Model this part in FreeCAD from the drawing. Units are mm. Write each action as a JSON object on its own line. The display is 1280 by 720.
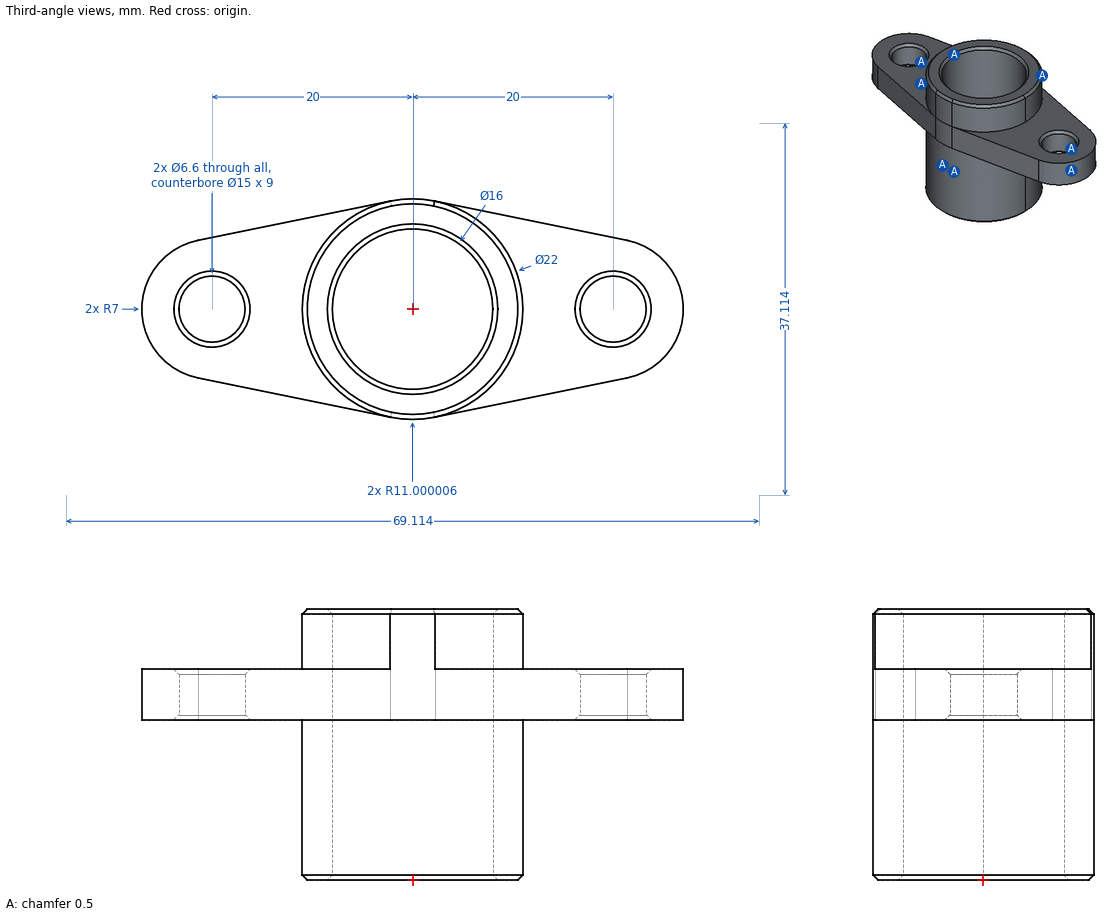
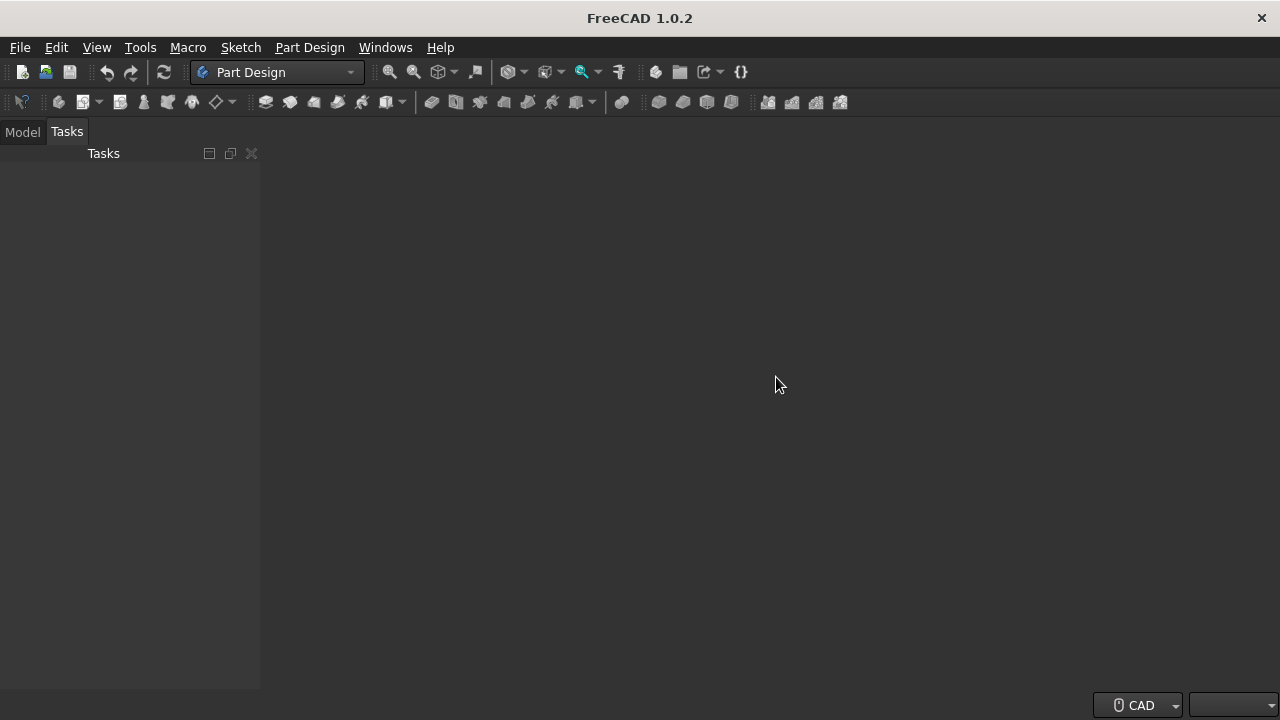
{"action": "left_click", "coordinate": [22, 72]}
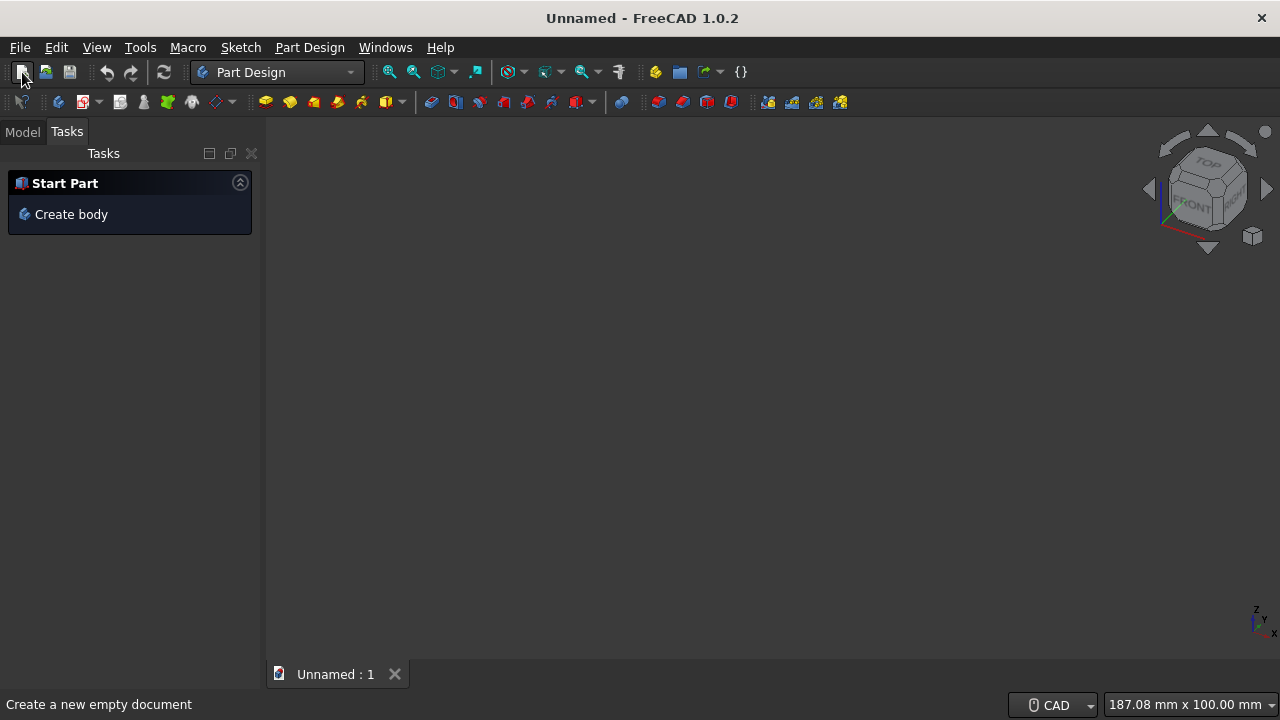
{"action": "left_click", "coordinate": [84, 102]}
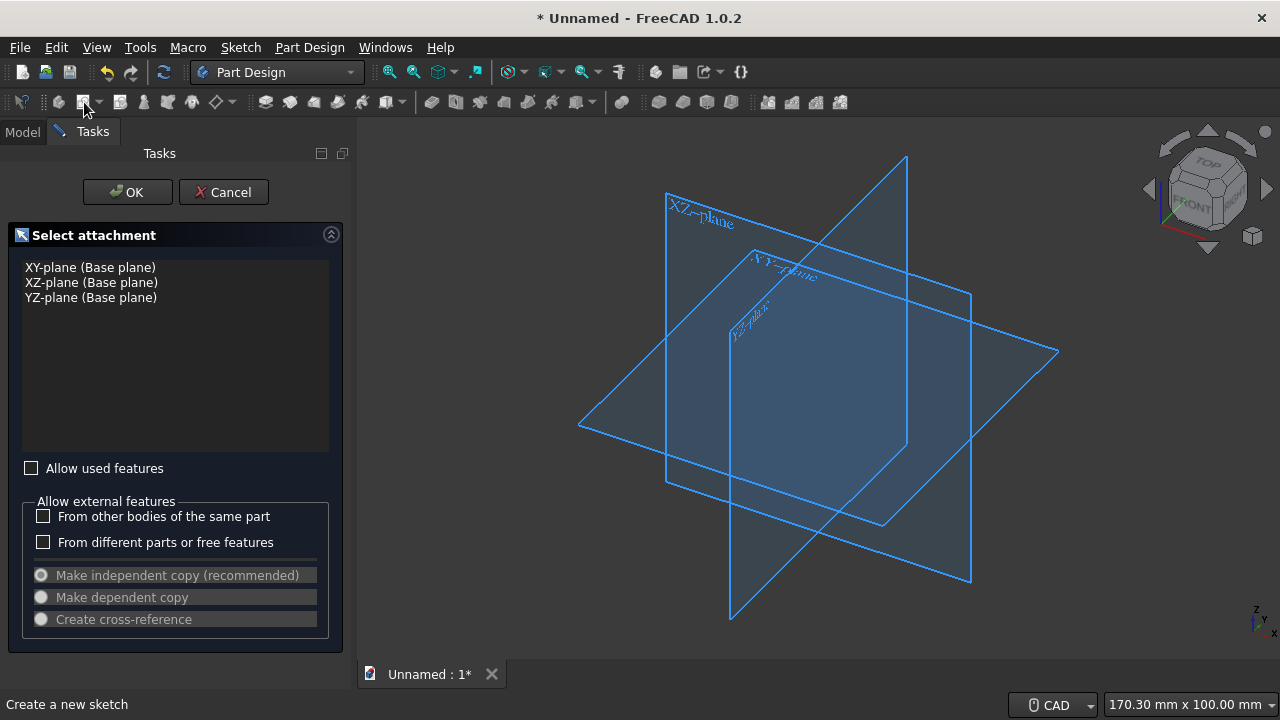
{"action": "left_click", "coordinate": [82, 268]}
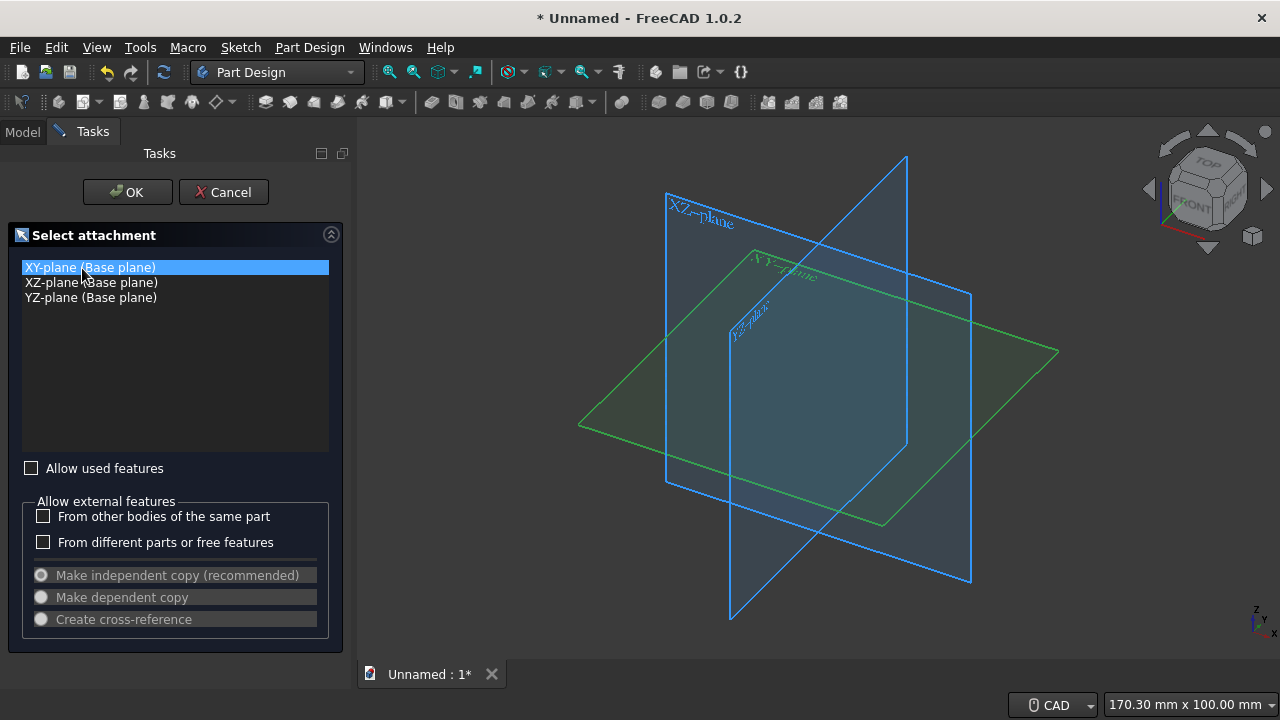
{"action": "left_click", "coordinate": [128, 192]}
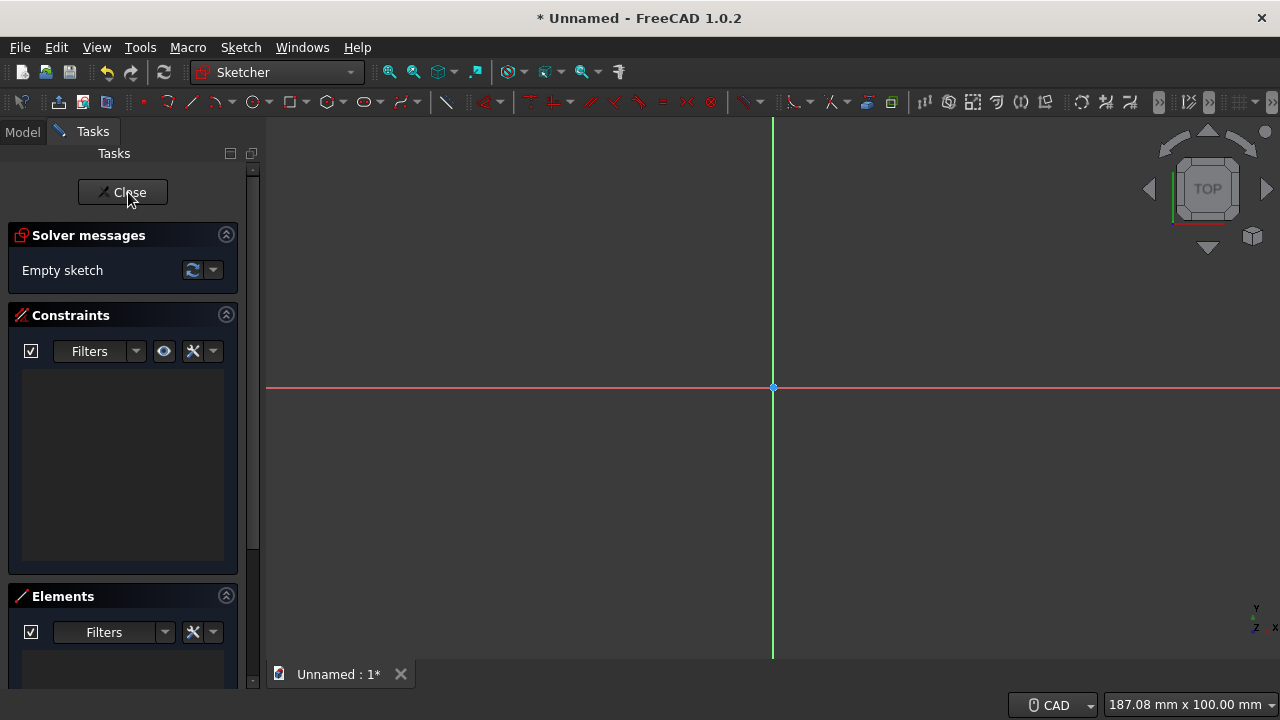
{"action": "scroll", "coordinate": [813, 388], "scroll_direction": "up", "scroll_amount": 5}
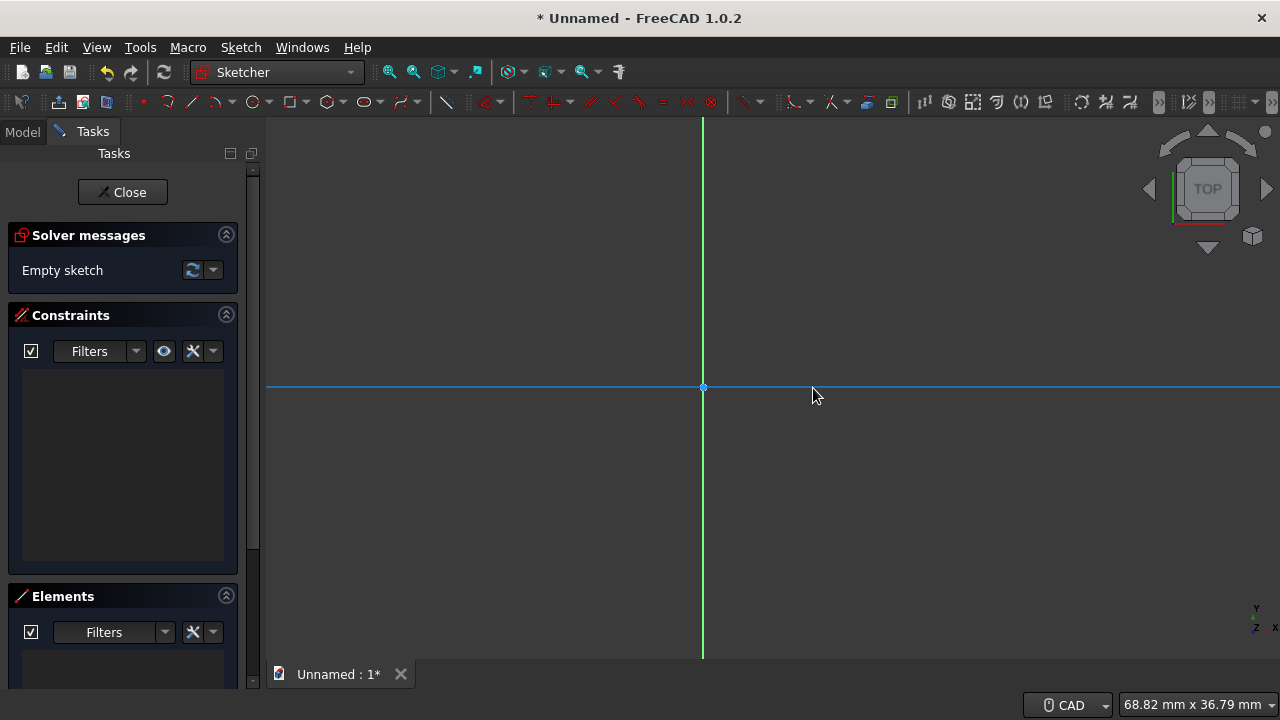
{"action": "left_click", "coordinate": [254, 102]}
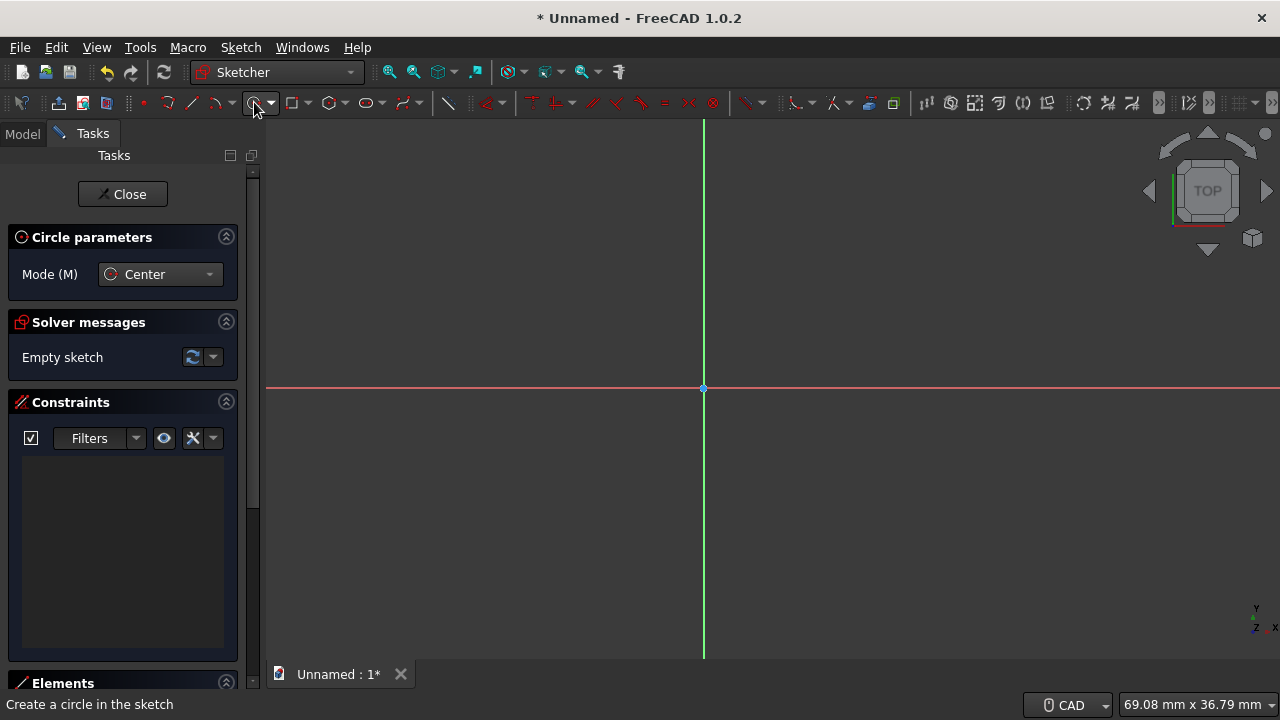
{"action": "left_click", "coordinate": [704, 388]}
{"action": "left_click", "coordinate": [818, 274]}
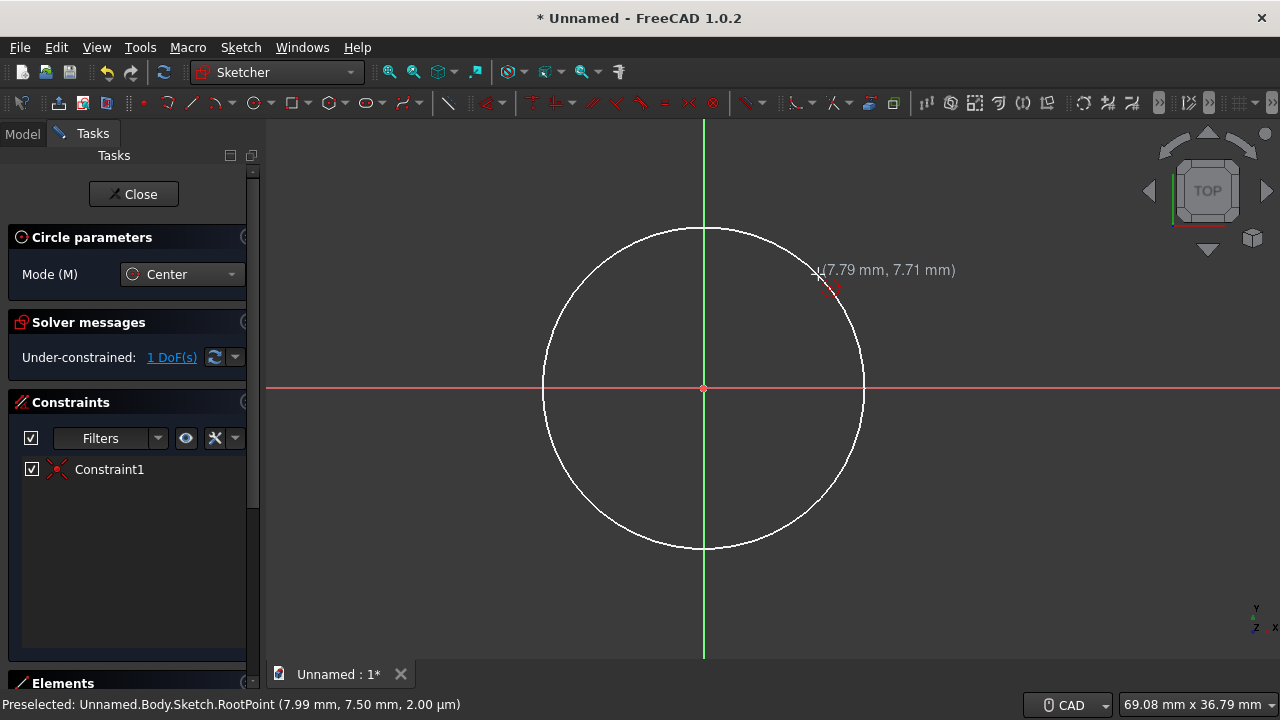
{"action": "left_click", "coordinate": [704, 388]}
{"action": "left_click", "coordinate": [787, 305]}
{"action": "key", "text": "Escape"}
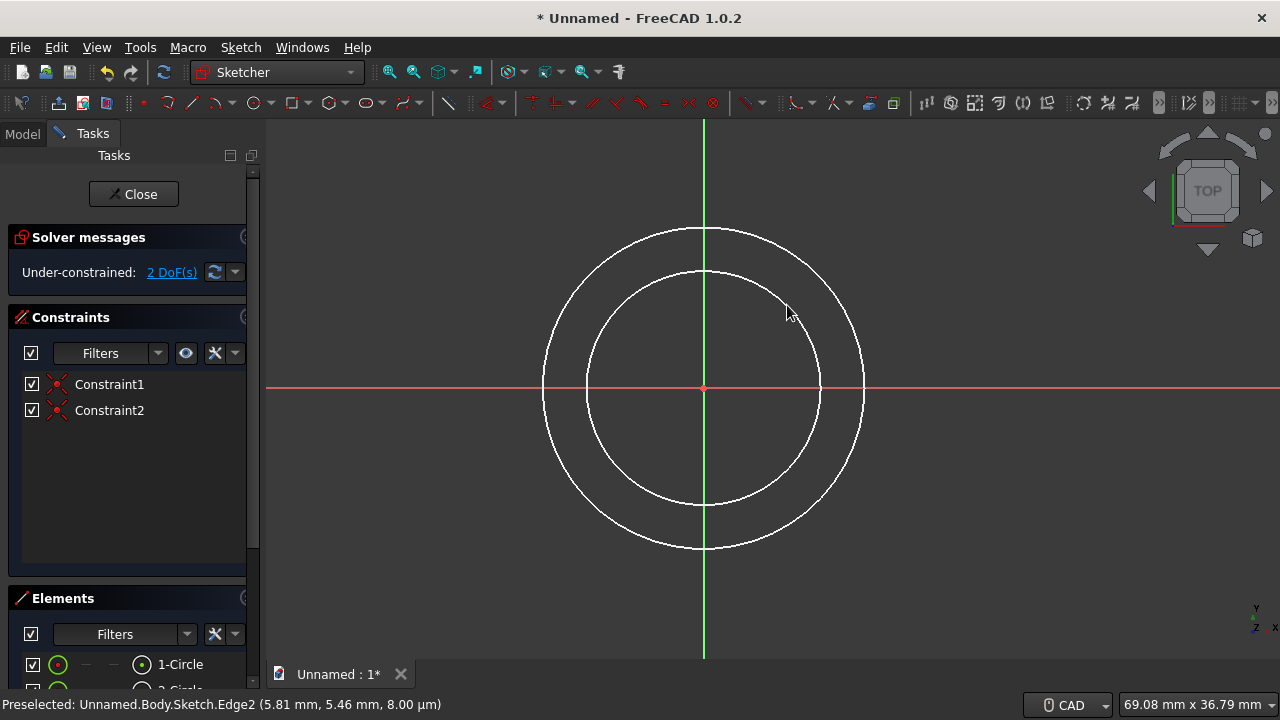
{"action": "left_click", "coordinate": [817, 274]}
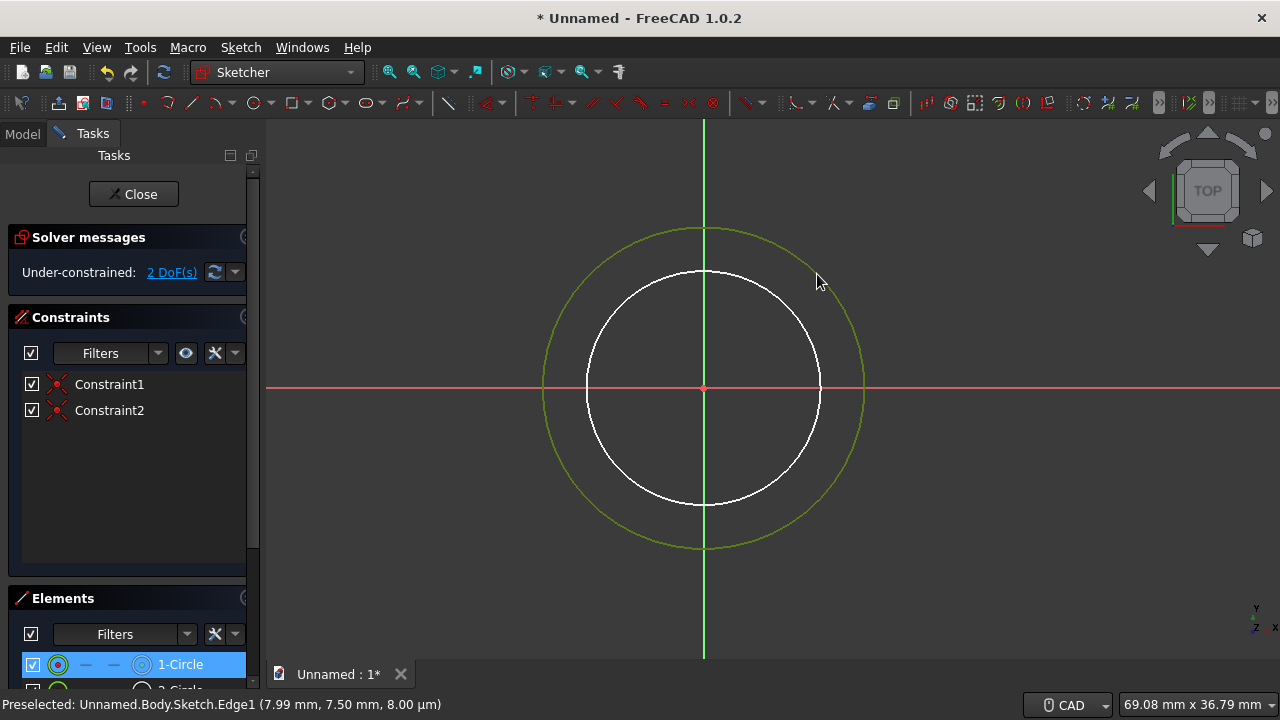
{"action": "left_click", "coordinate": [504, 104]}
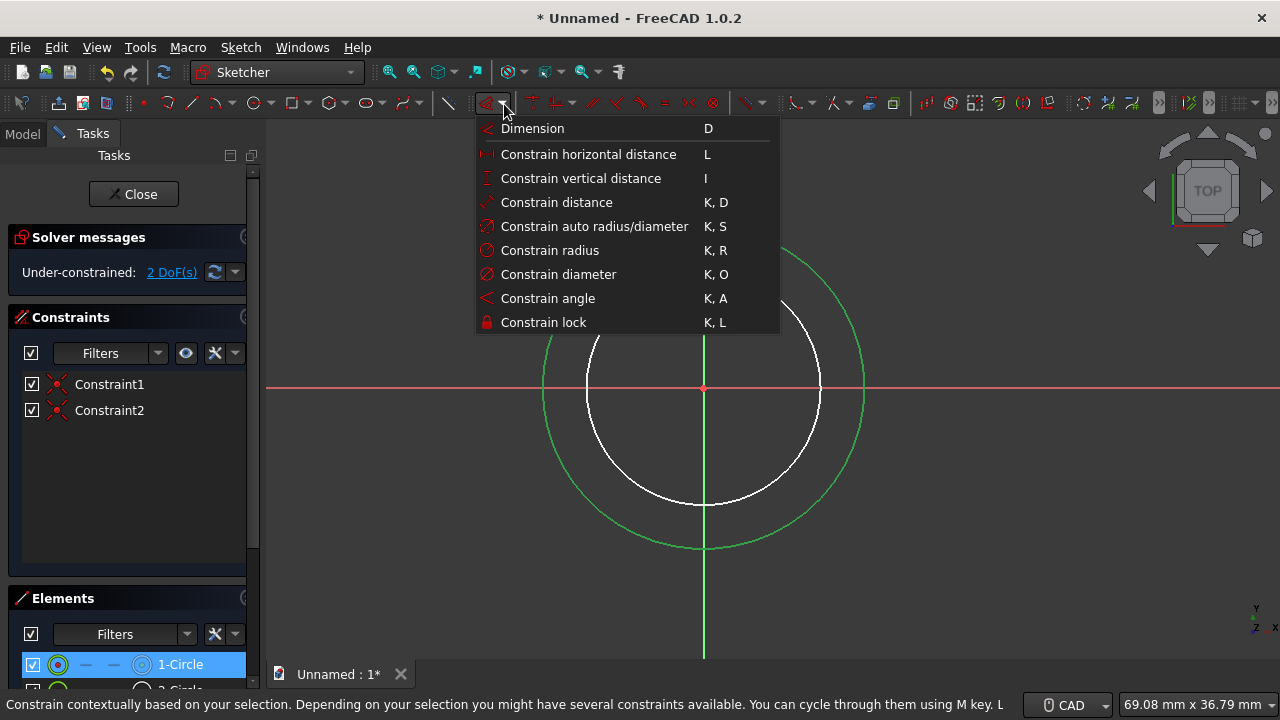
{"action": "left_click", "coordinate": [628, 274]}